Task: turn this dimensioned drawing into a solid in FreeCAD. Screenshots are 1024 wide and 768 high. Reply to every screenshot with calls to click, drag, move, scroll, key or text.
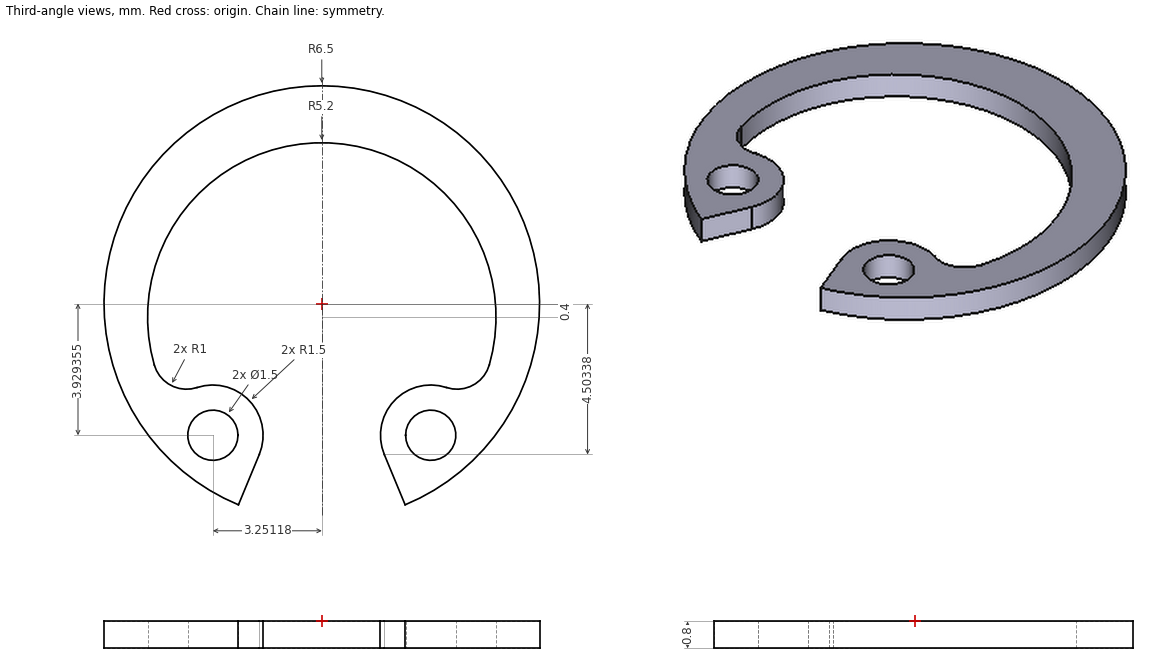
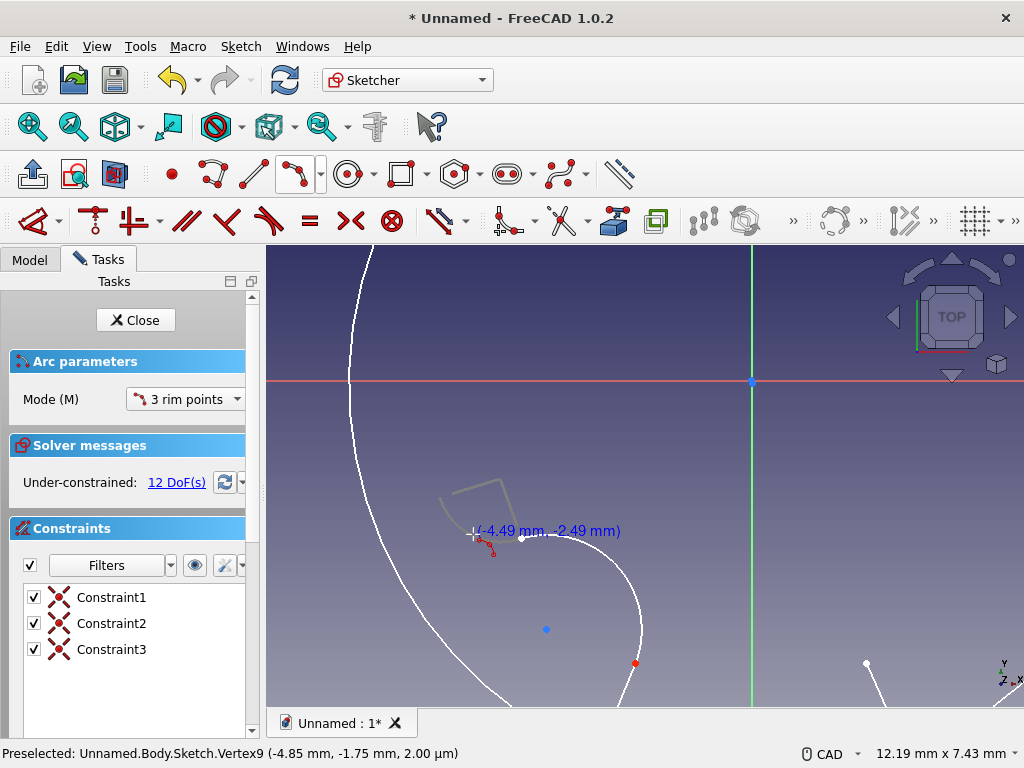
click(472, 532)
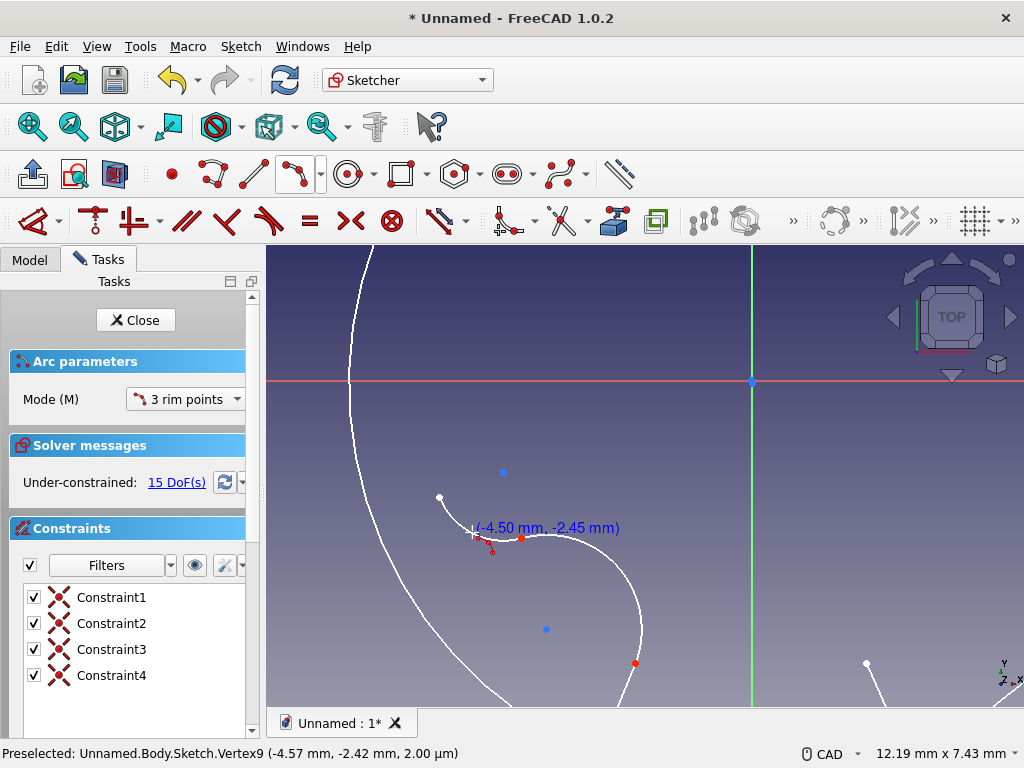
click(440, 498)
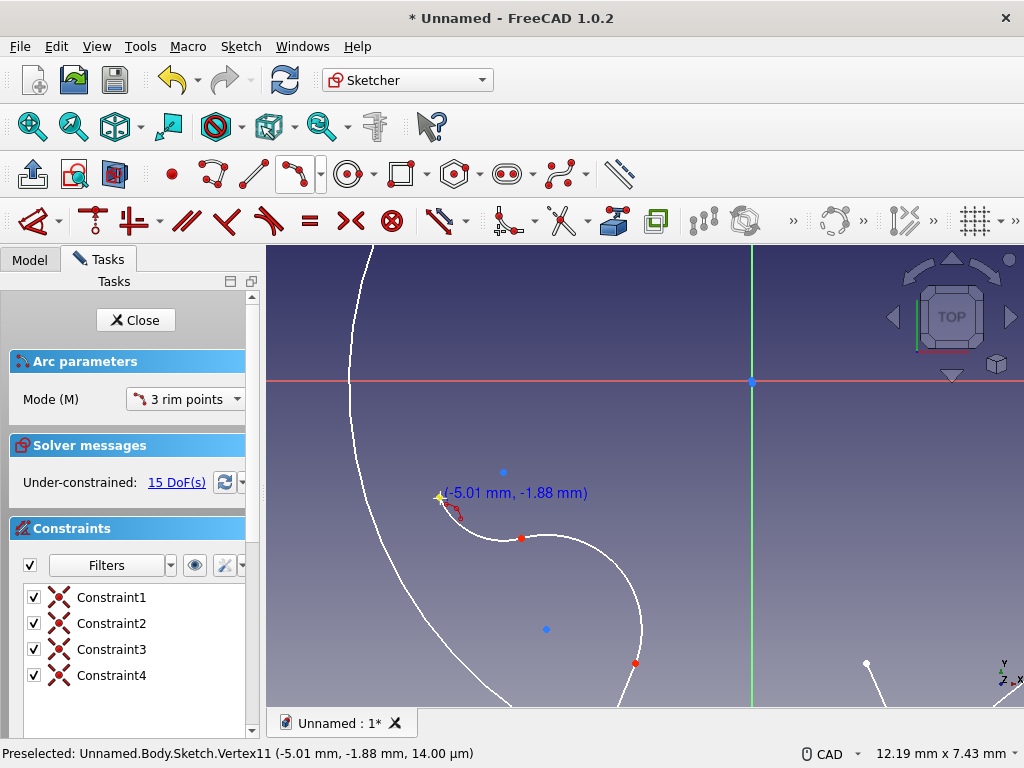
scroll(474, 540, down, 5)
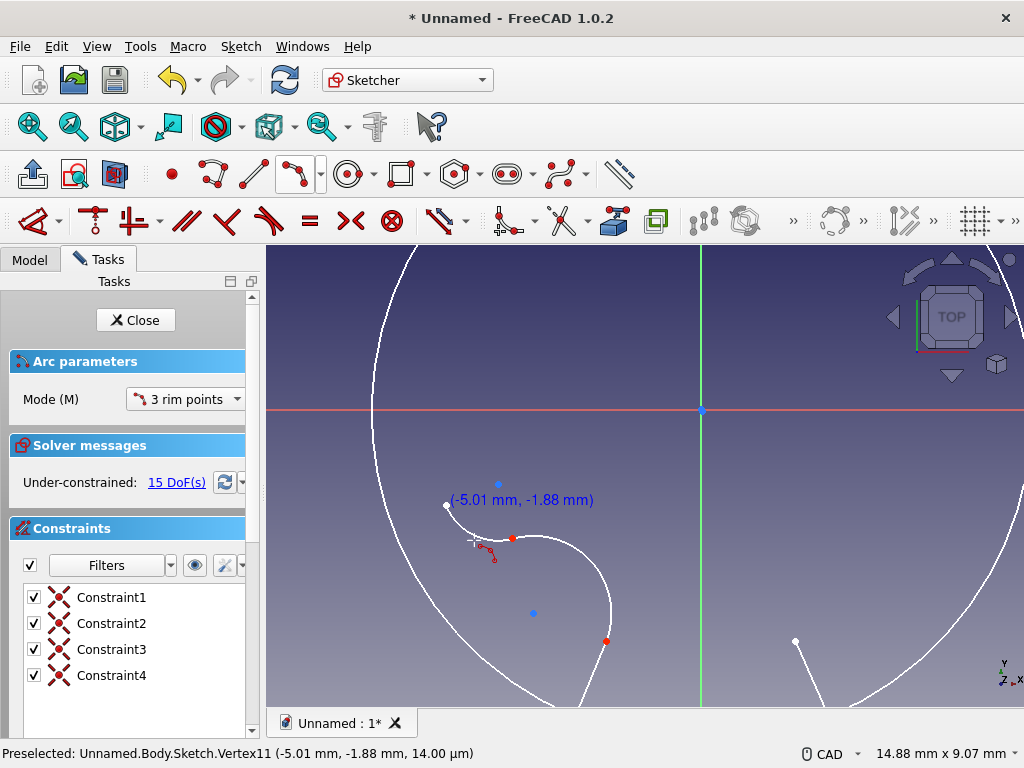
click(691, 524)
click(619, 380)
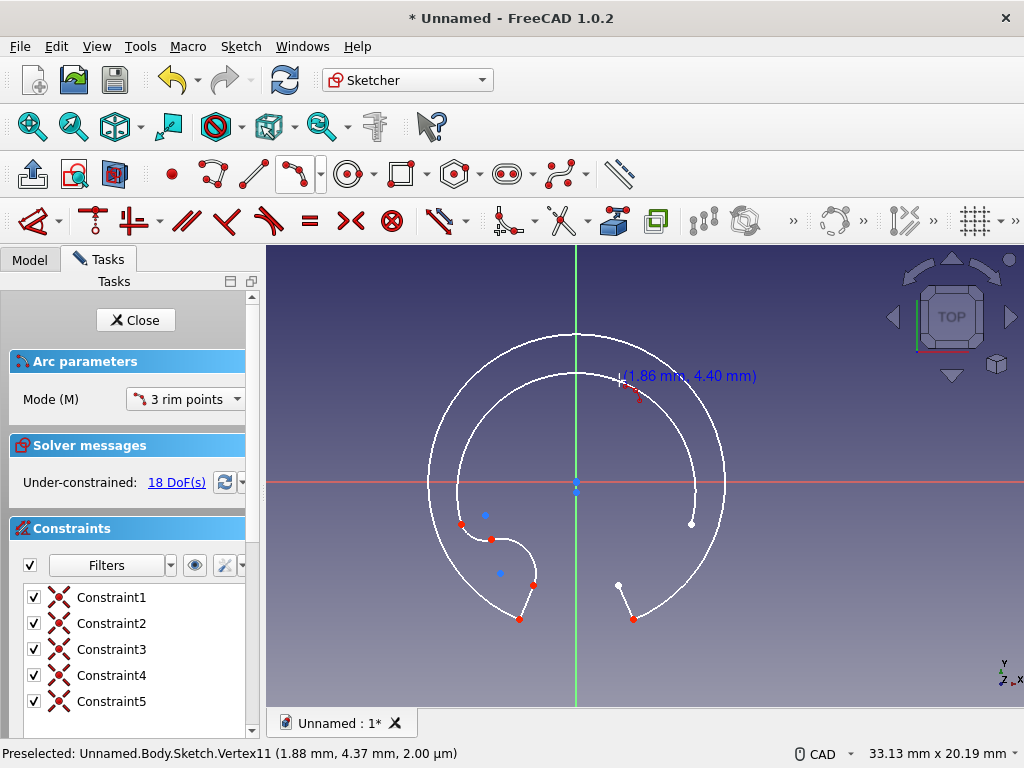
click(691, 525)
click(662, 539)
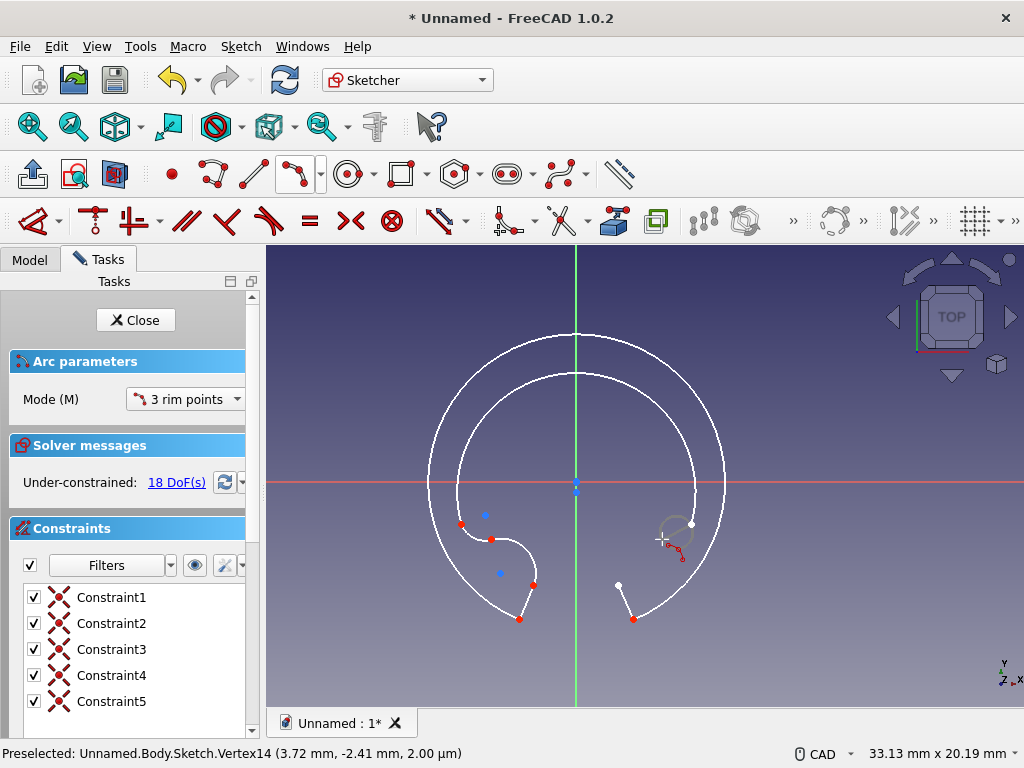
scroll(679, 538, up, 5)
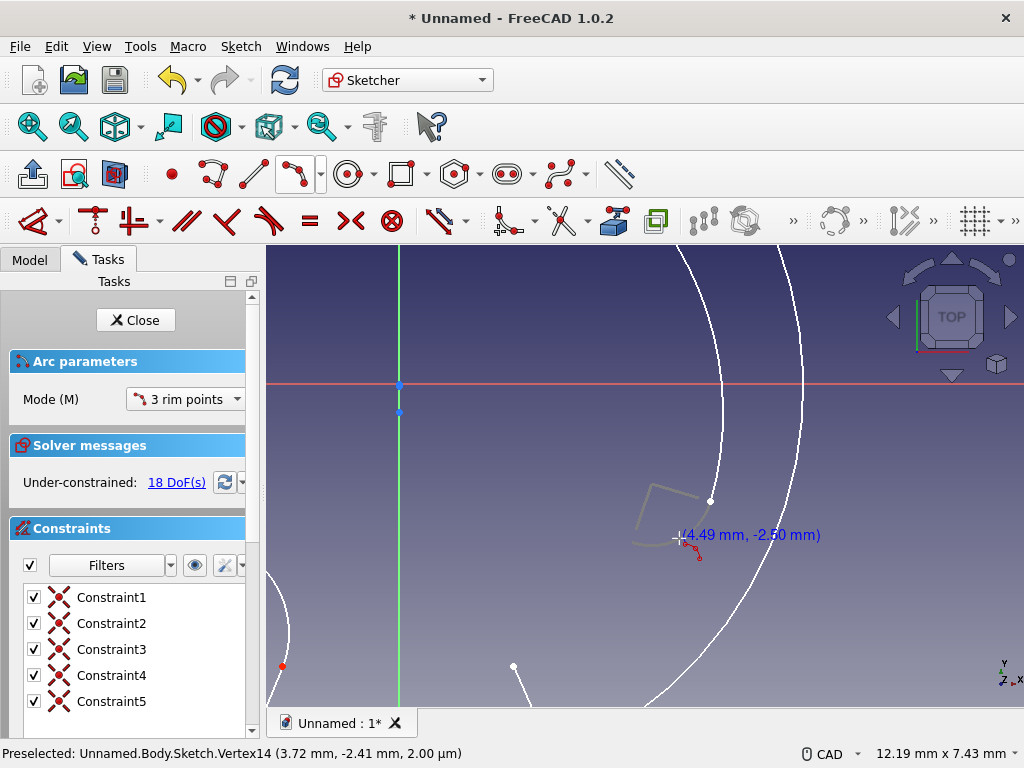
click(679, 536)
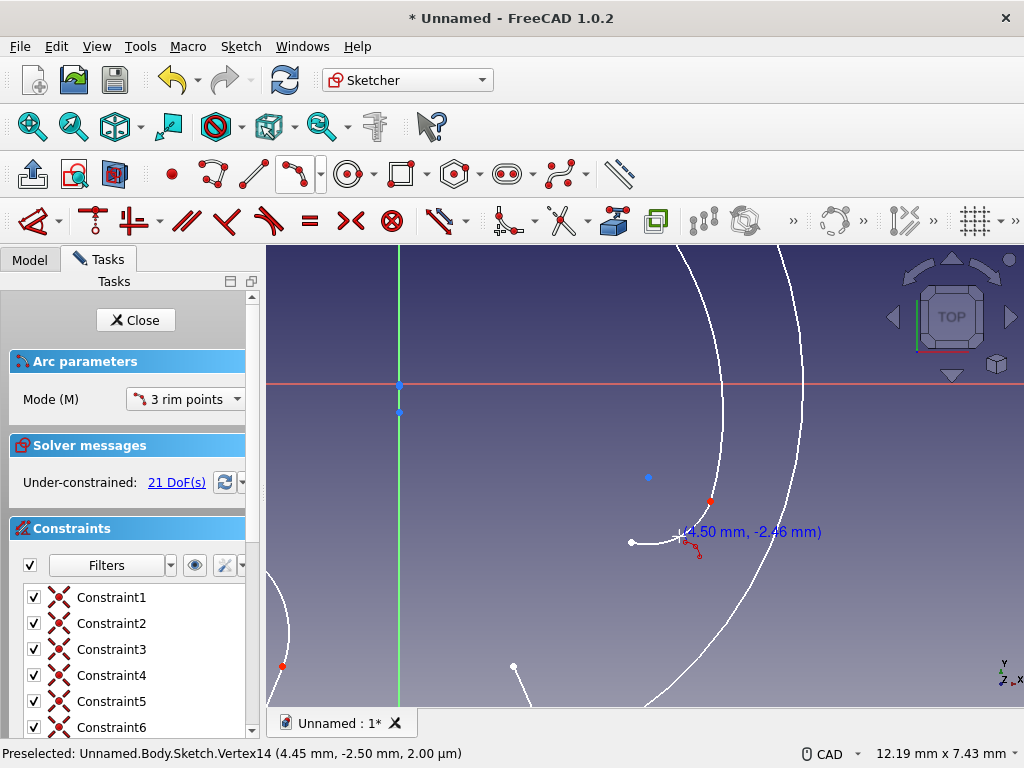
click(632, 542)
click(514, 667)
click(533, 565)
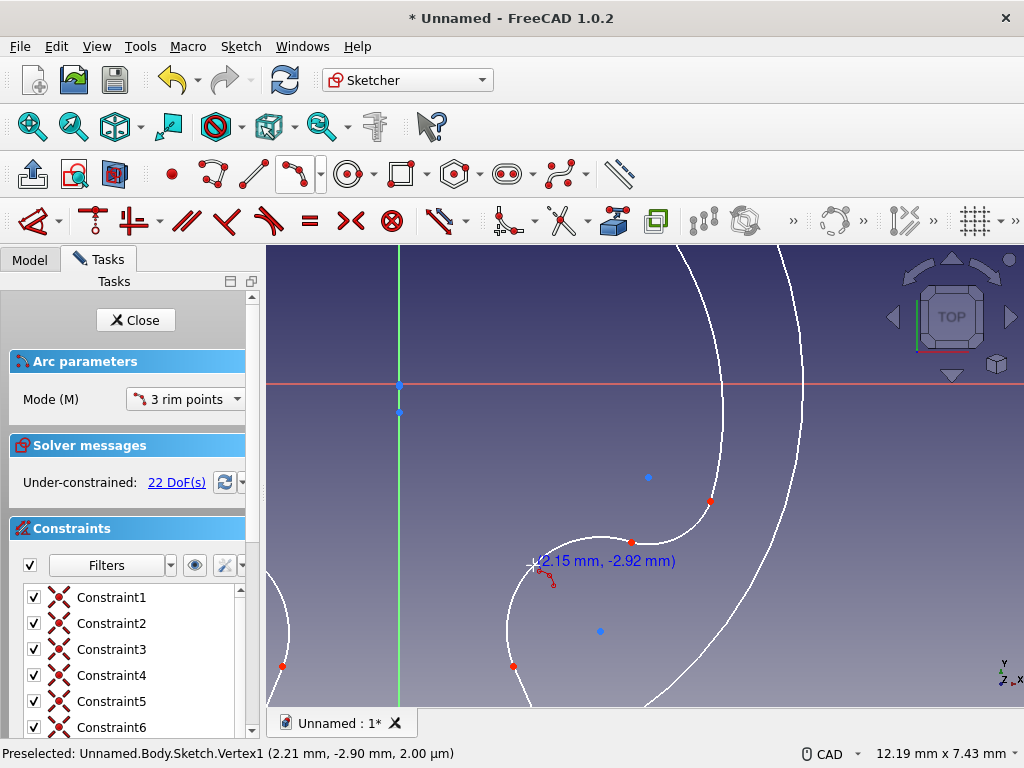
click(348, 174)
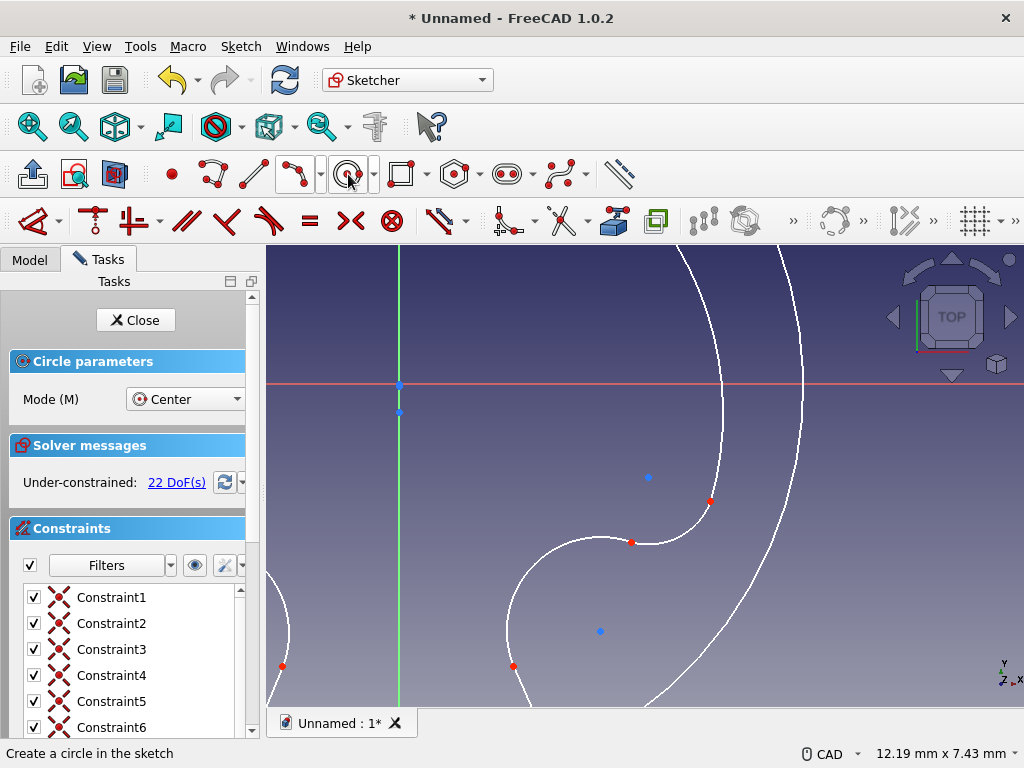
scroll(680, 538, down, 5)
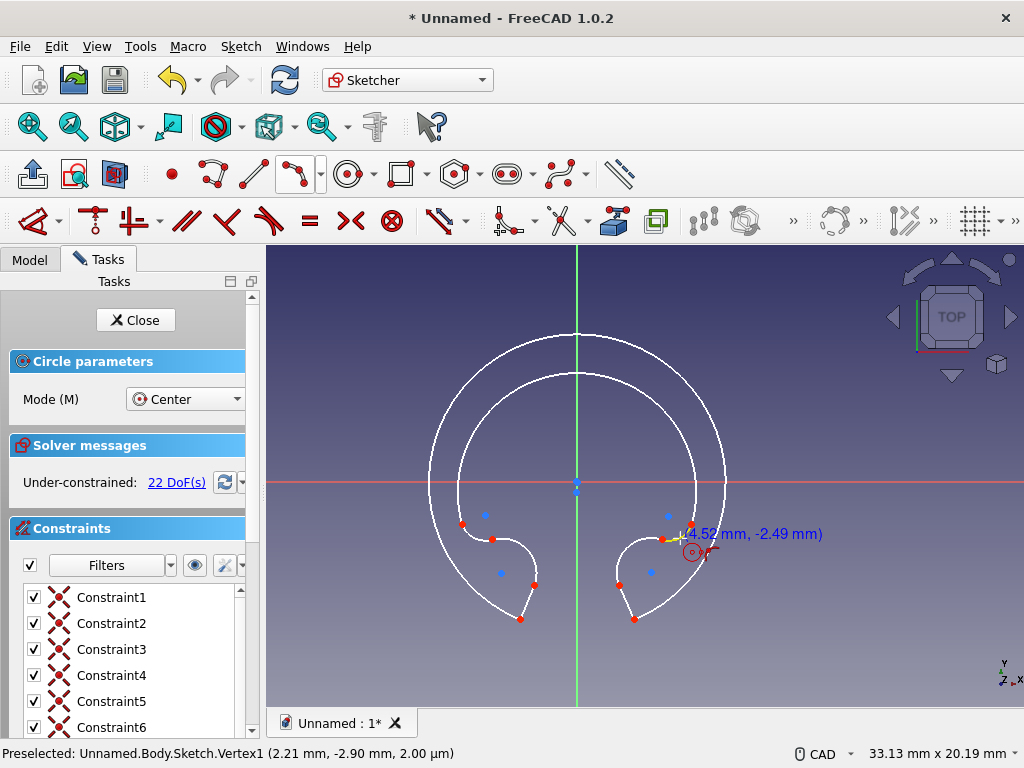
scroll(503, 572, up, 2)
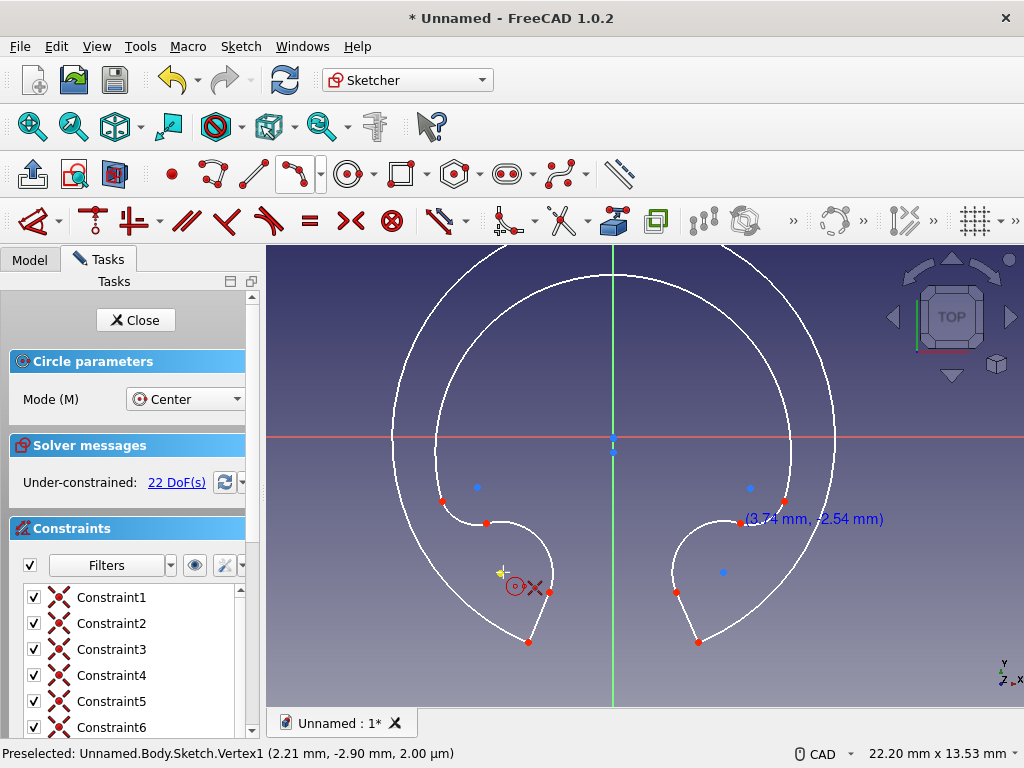
click(502, 571)
move(520, 553)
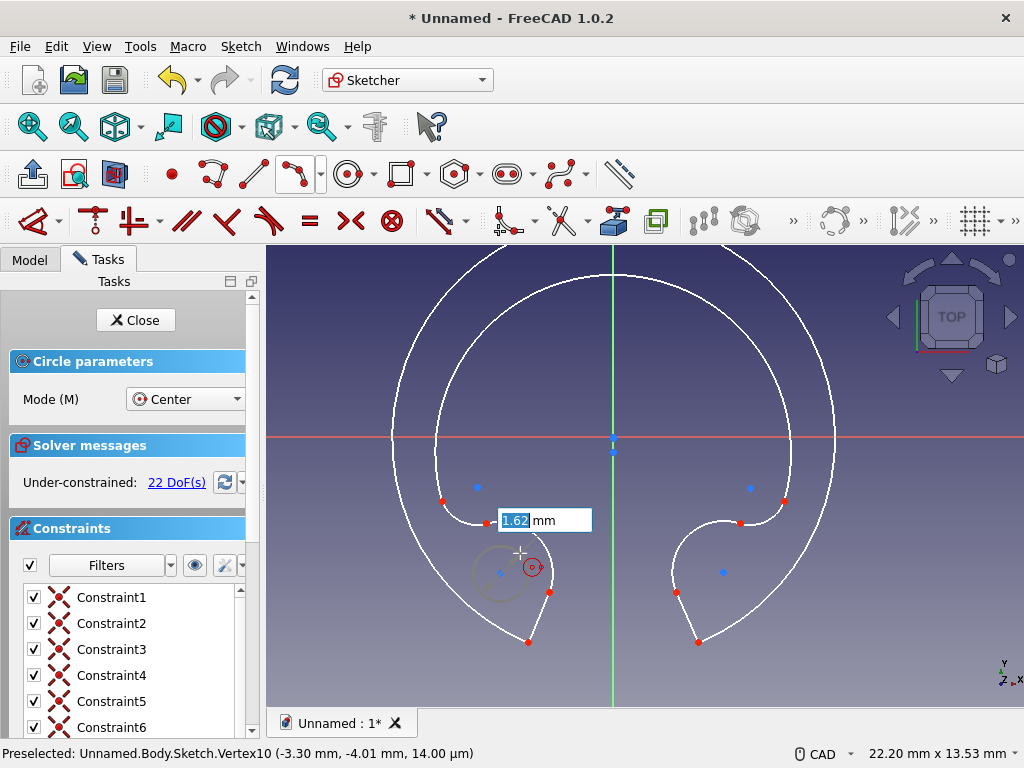
text(1.5)
key(Return)